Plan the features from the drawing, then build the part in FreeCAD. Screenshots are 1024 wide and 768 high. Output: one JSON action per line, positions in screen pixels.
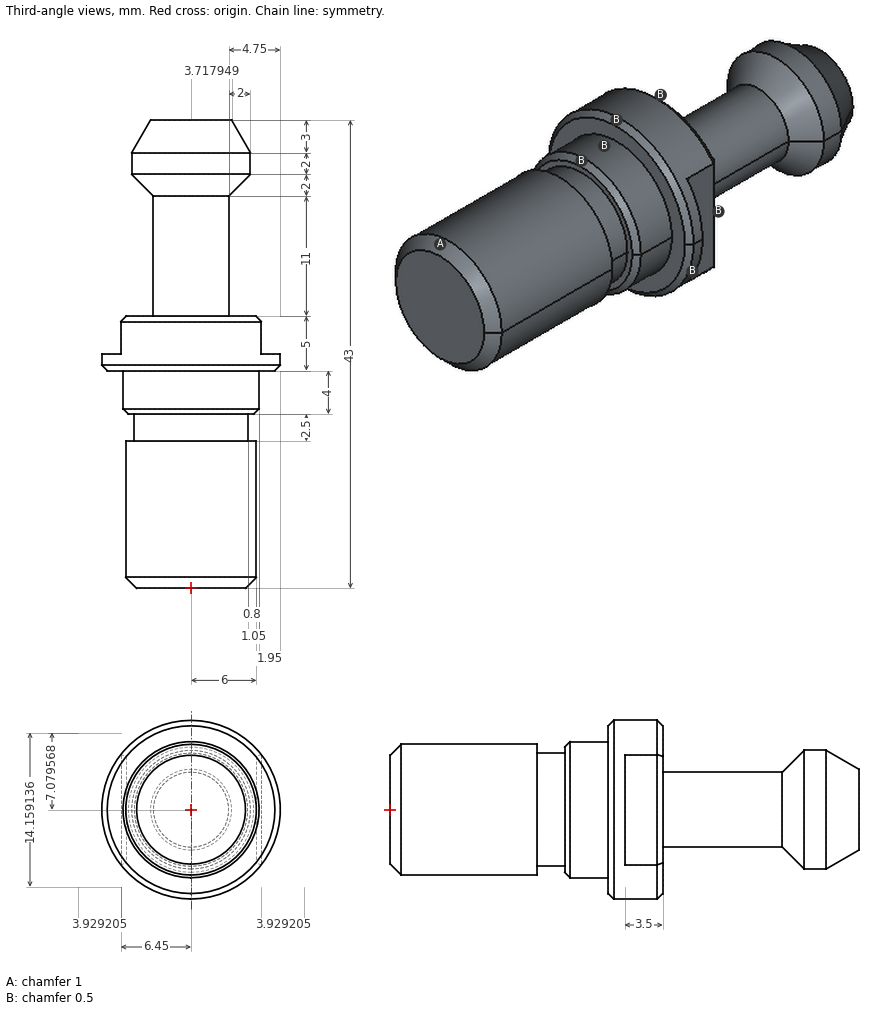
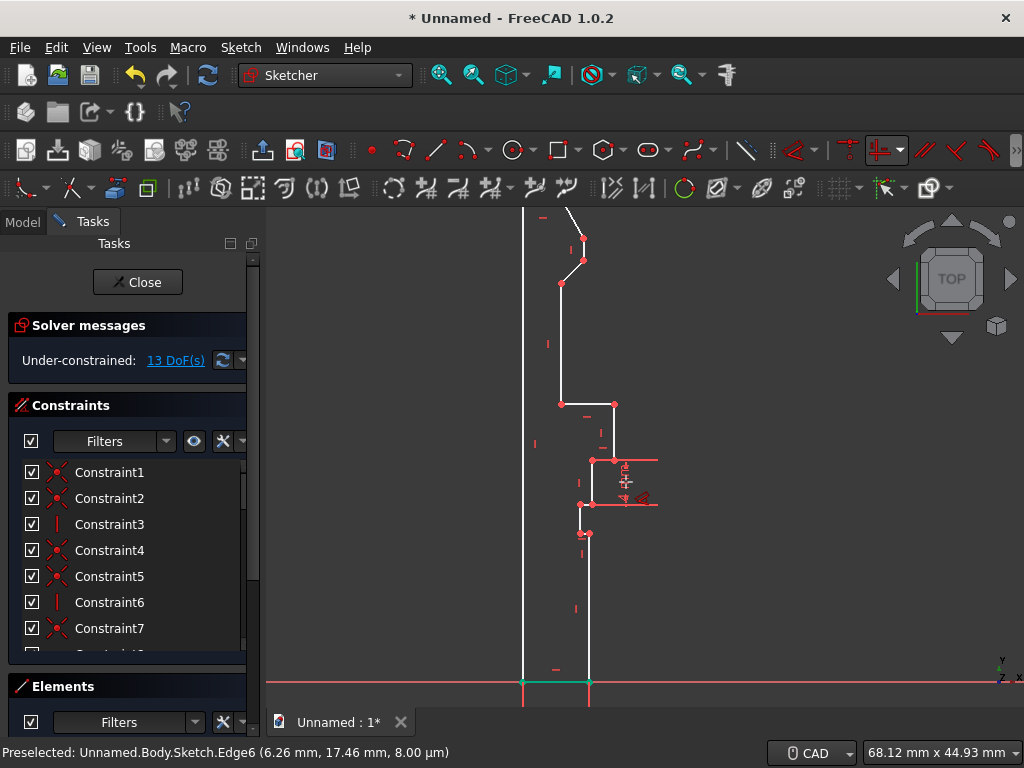
{"action": "left_click", "coordinate": [614, 444]}
{"action": "left_click", "coordinate": [648, 432]}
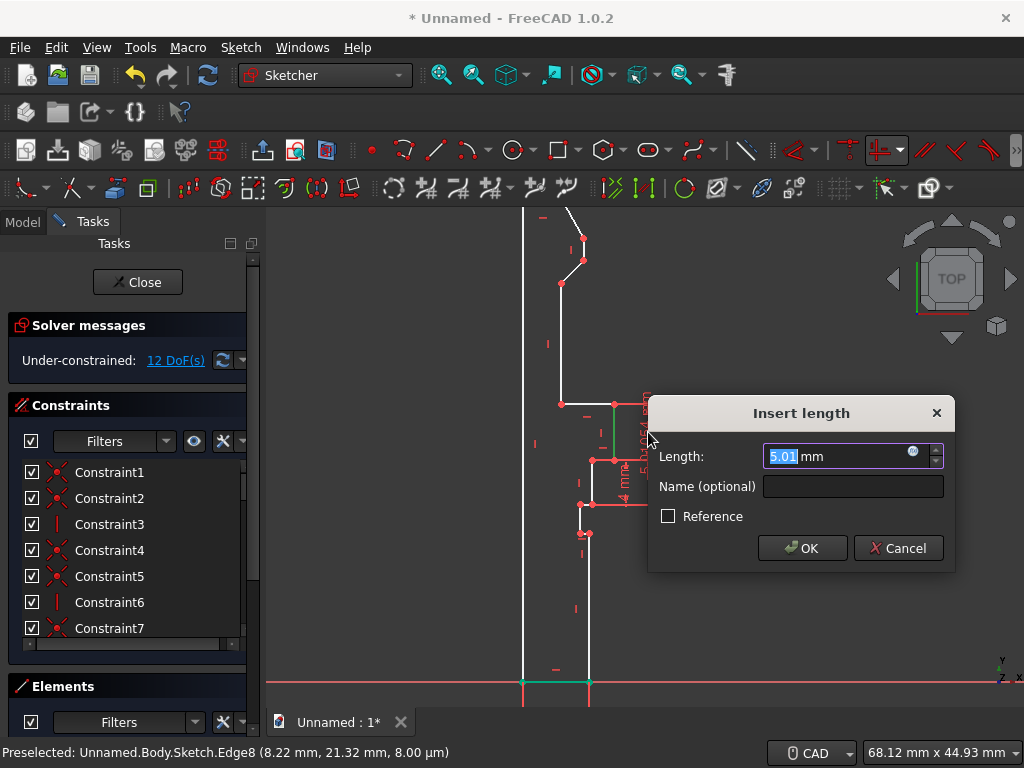
{"action": "type", "text": "5"}
{"action": "key", "text": "Return"}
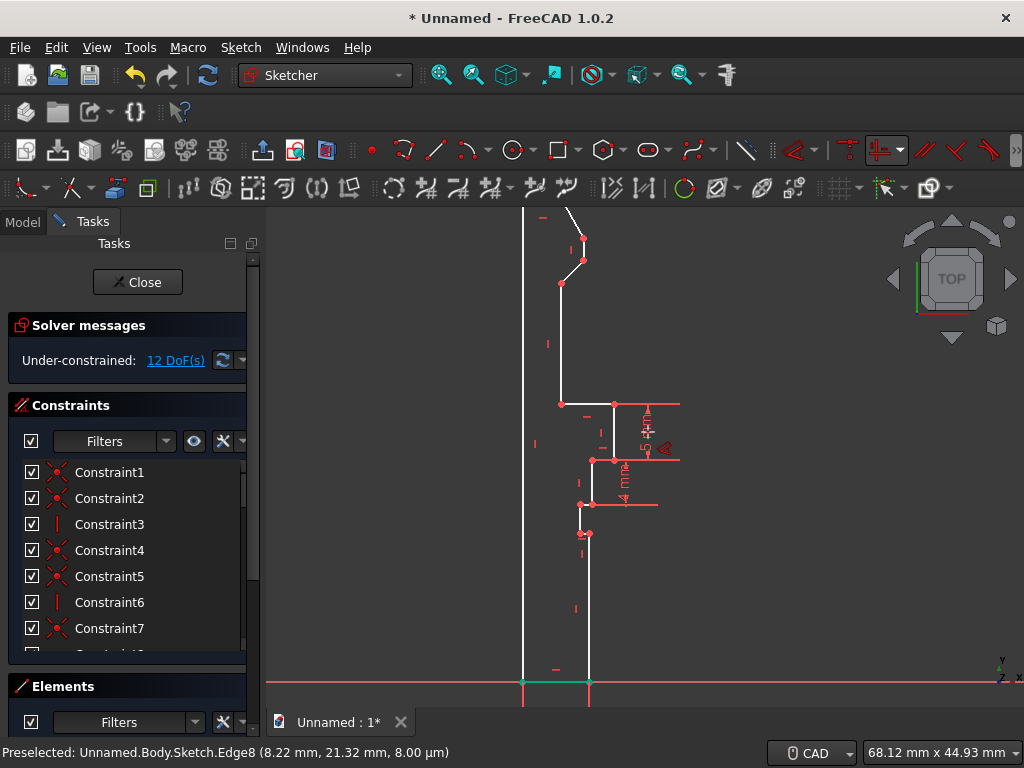
{"action": "scroll", "coordinate": [584, 250], "scroll_direction": "up", "scroll_amount": 3}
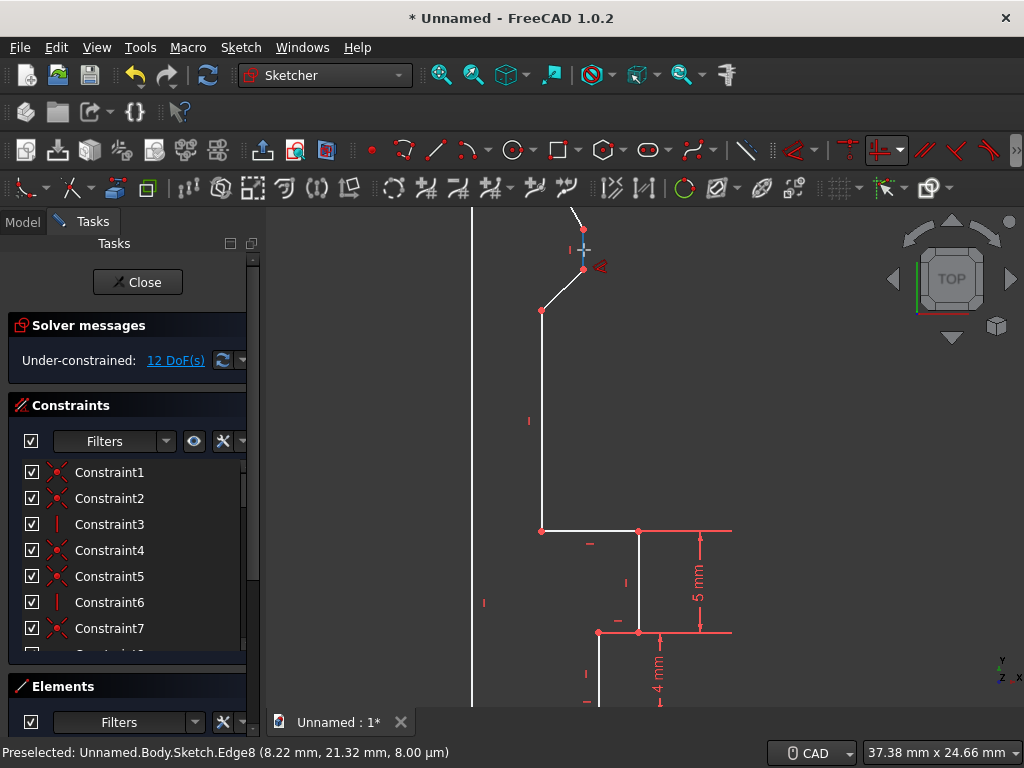
{"action": "left_click", "coordinate": [583, 250]}
{"action": "left_click", "coordinate": [617, 252]}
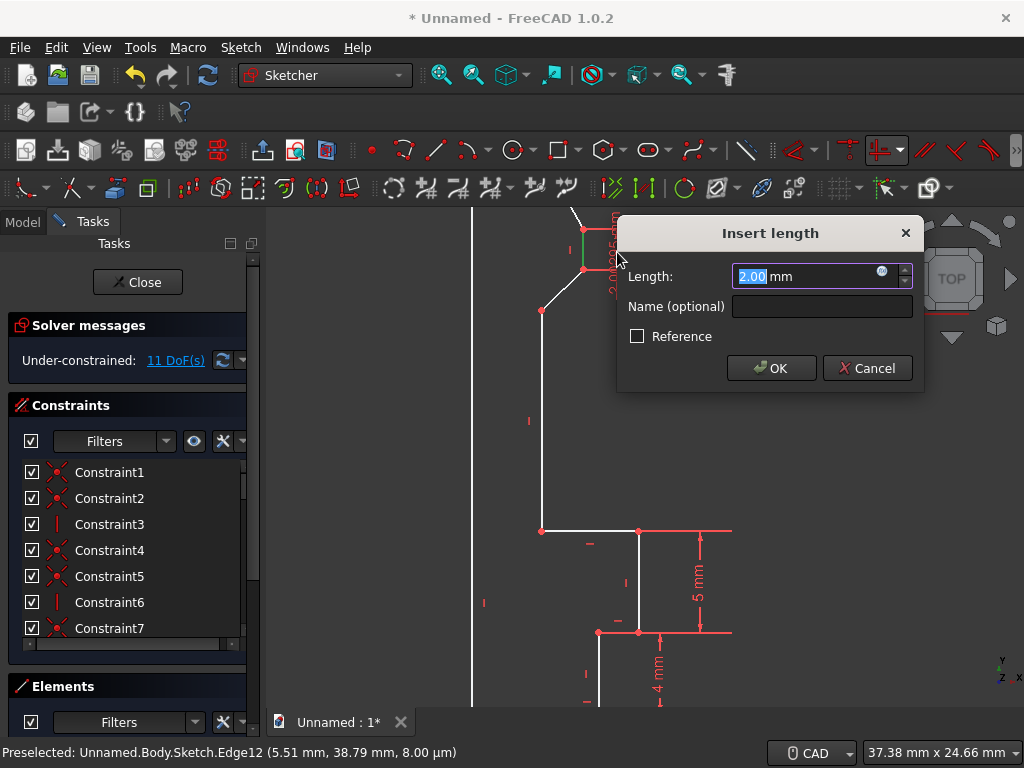
{"action": "type", "text": "2"}
{"action": "key", "text": "Return"}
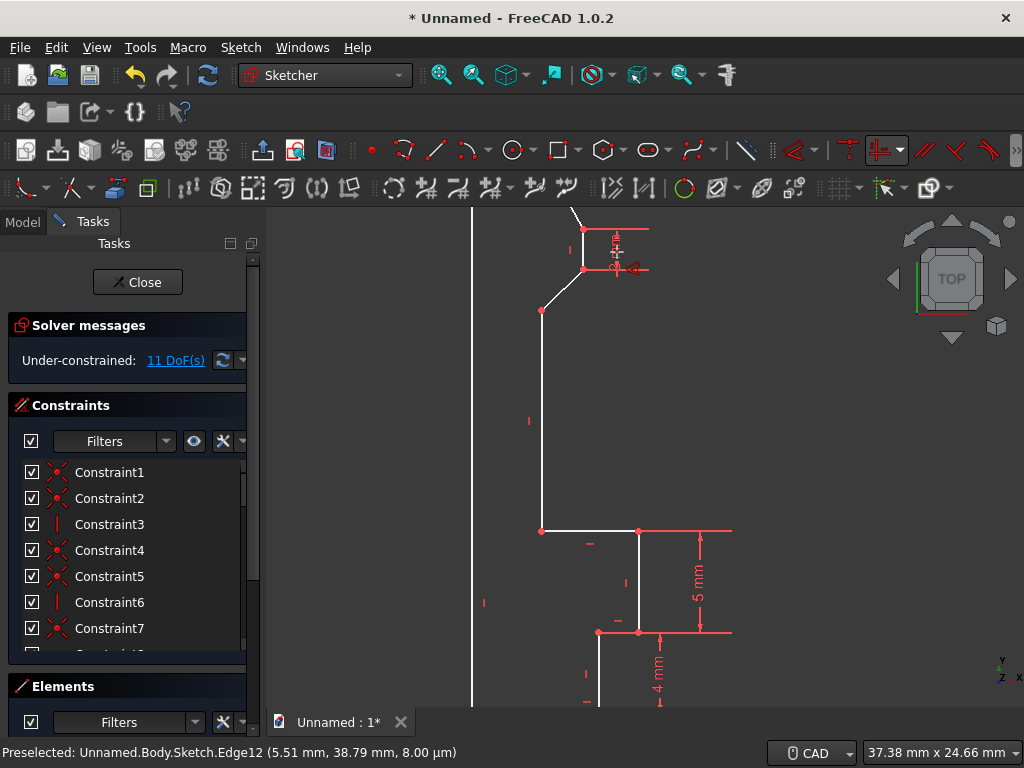
{"action": "left_click", "coordinate": [542, 465]}
{"action": "left_click", "coordinate": [508, 421]}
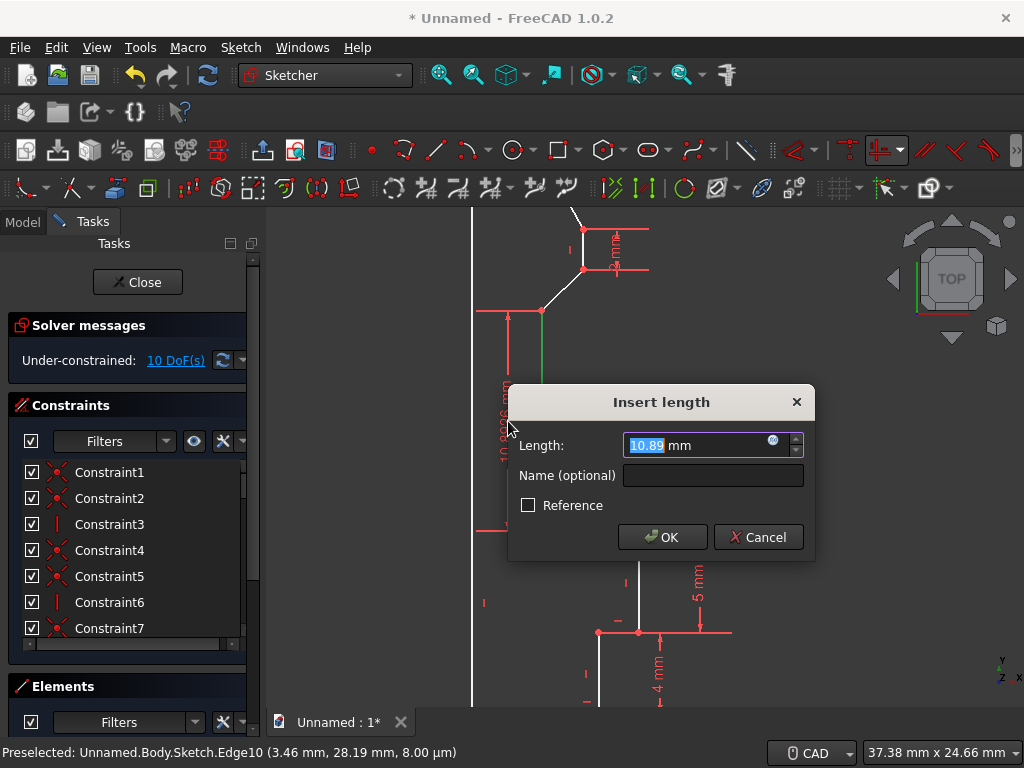
{"action": "type", "text": "11"}
{"action": "key", "text": "Return"}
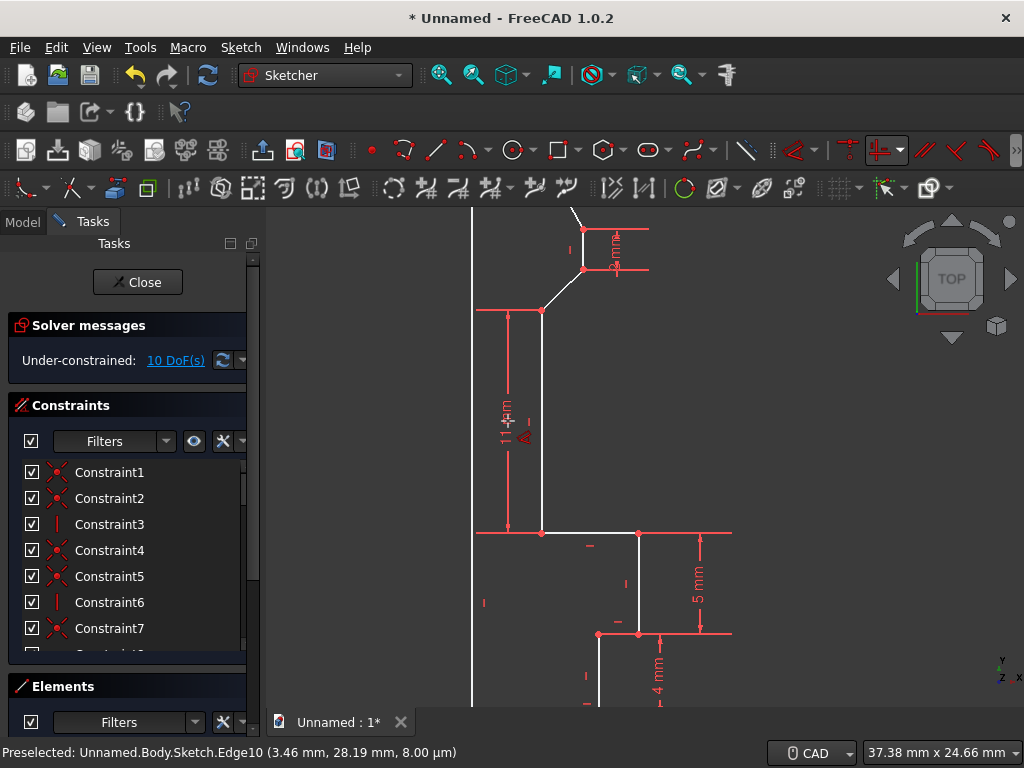
{"action": "left_click", "coordinate": [472, 428]}
{"action": "left_click", "coordinate": [438, 457]}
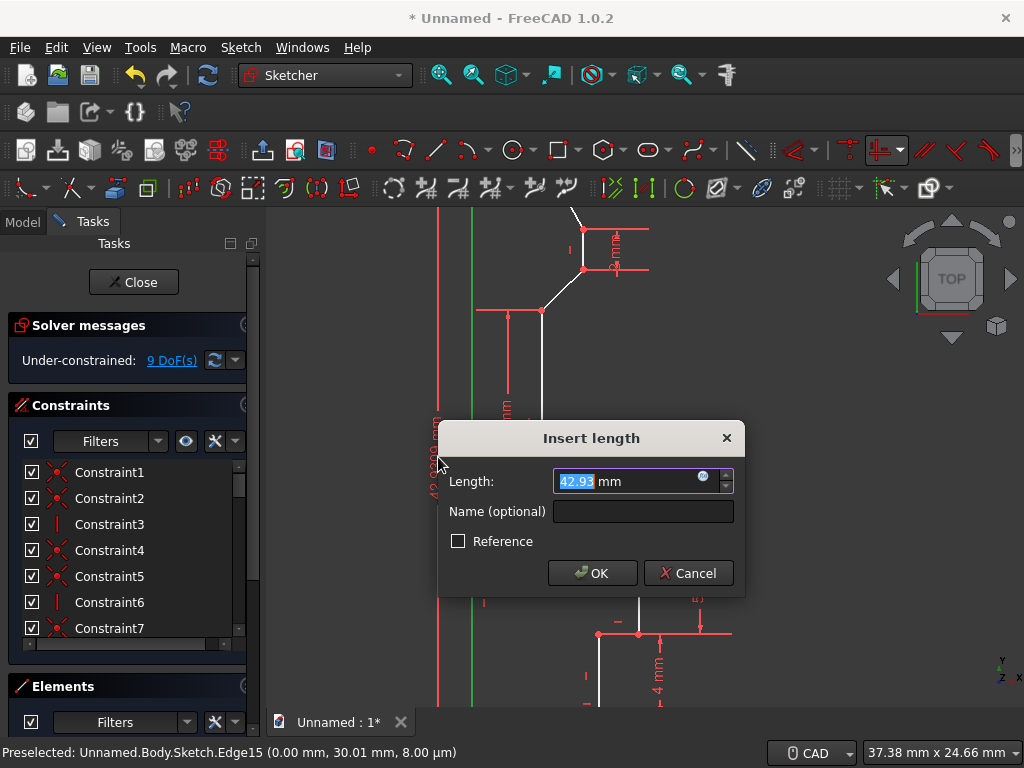
{"action": "type", "text": "43"}
{"action": "key", "text": "Return"}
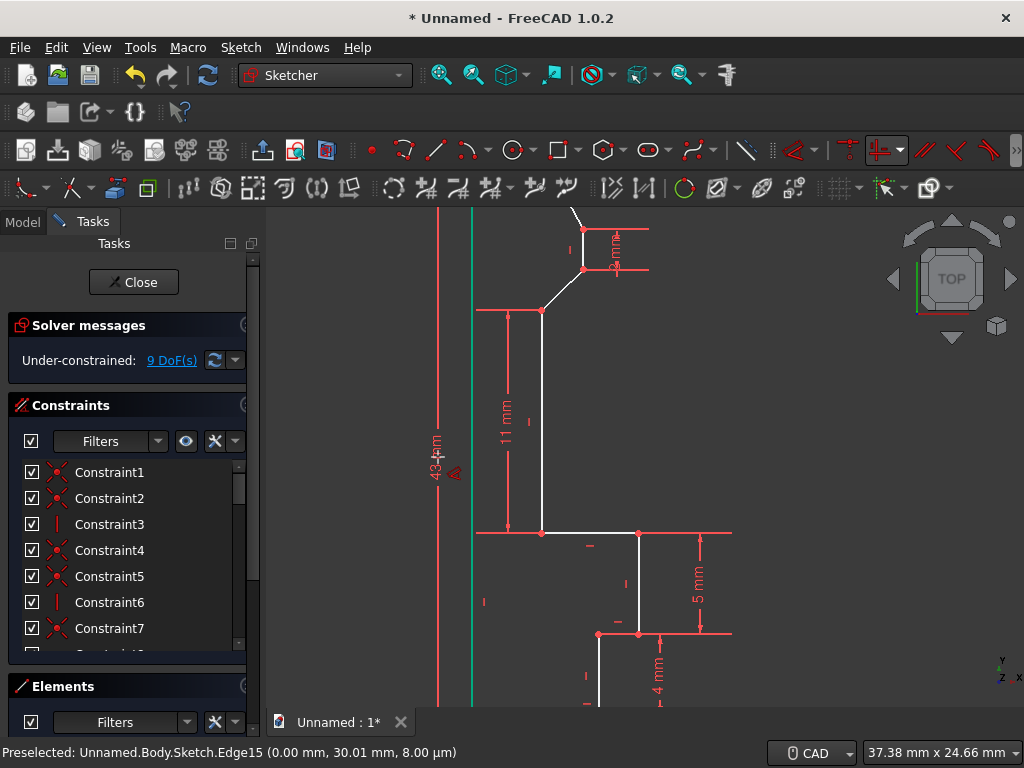
{"action": "left_click", "coordinate": [554, 298]}
{"action": "left_click", "coordinate": [563, 344]}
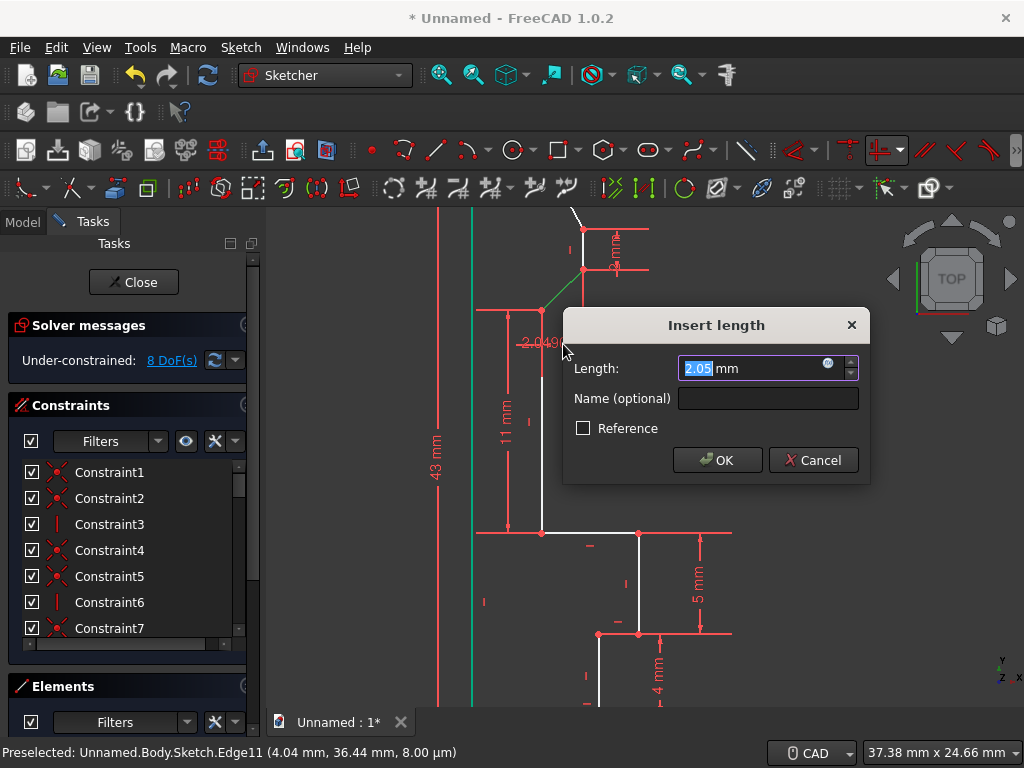
{"action": "type", "text": "2"}
{"action": "key", "text": "Return"}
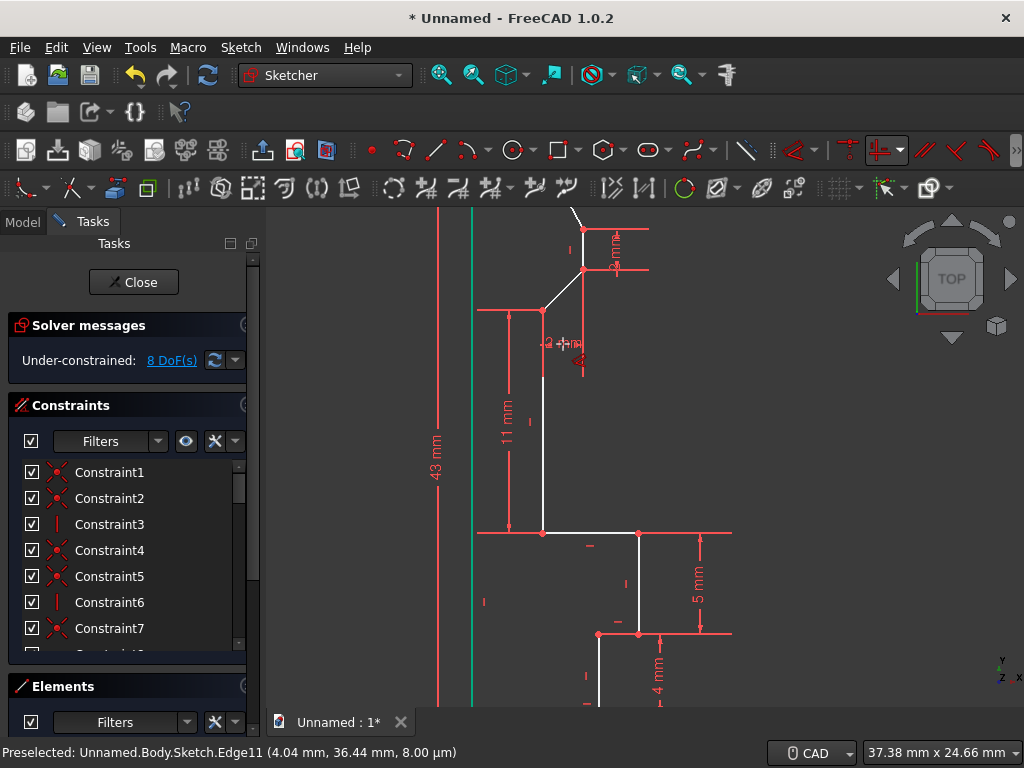
{"action": "left_click", "coordinate": [555, 298]}
{"action": "left_click", "coordinate": [617, 290]}